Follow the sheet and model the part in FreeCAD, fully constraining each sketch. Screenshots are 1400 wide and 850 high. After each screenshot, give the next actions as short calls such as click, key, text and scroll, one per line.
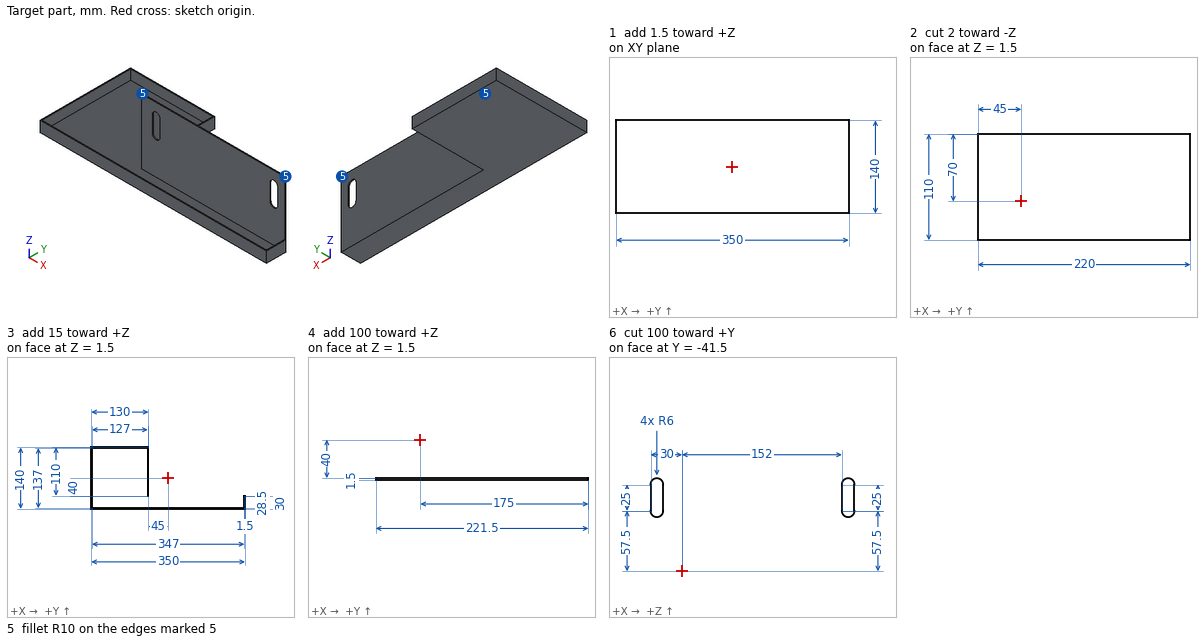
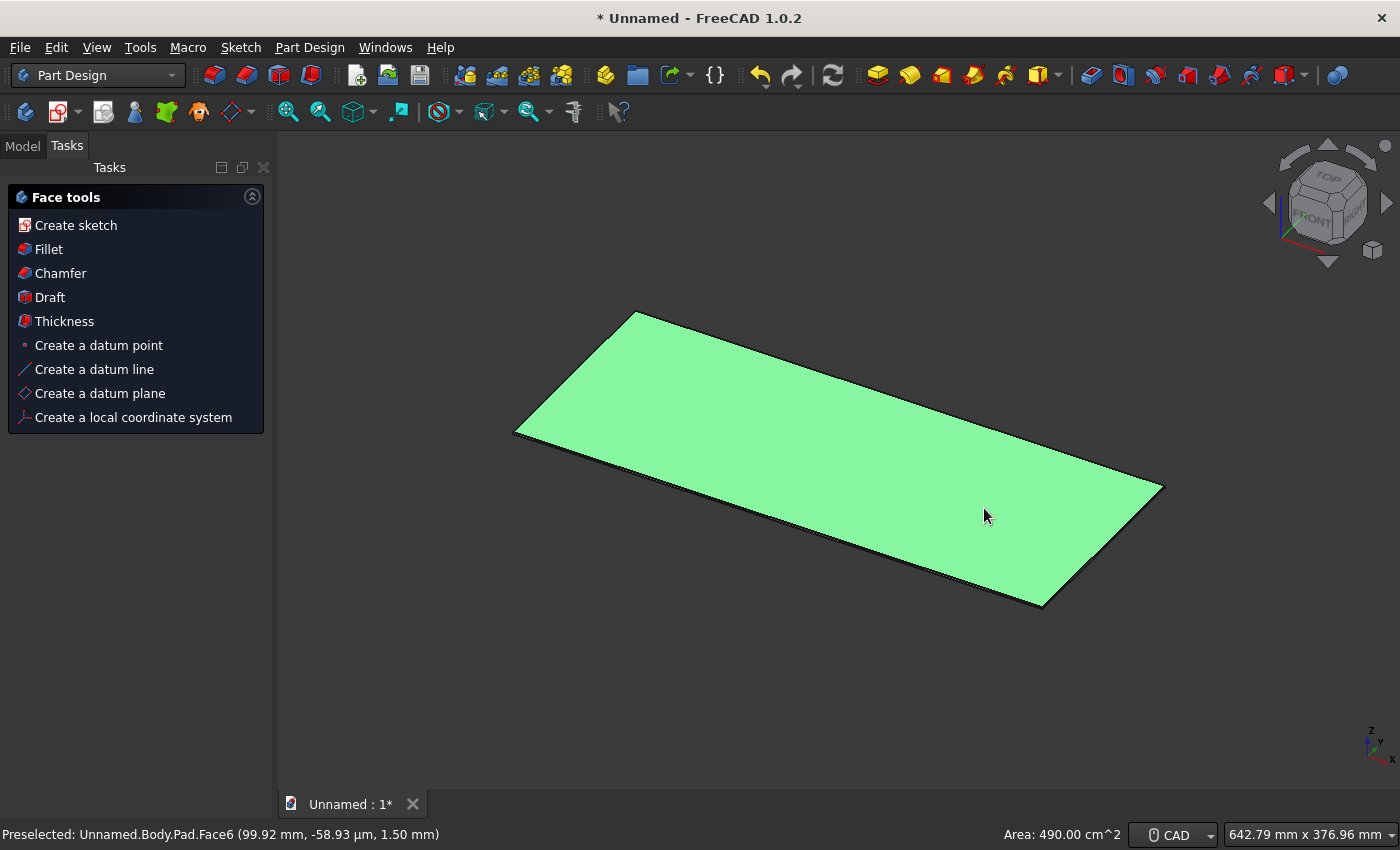
click(58, 112)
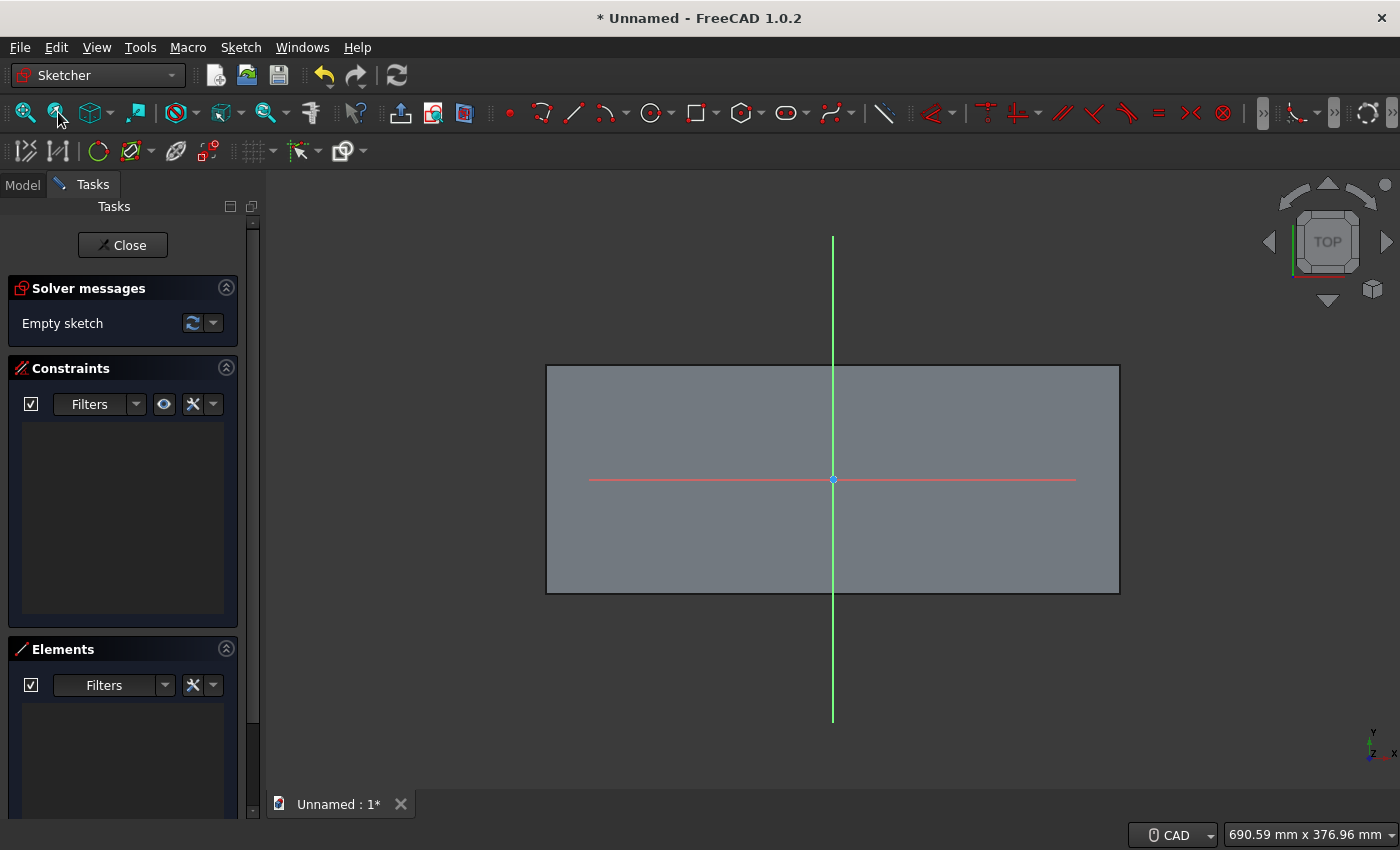
scroll(1153, 425, up, 3)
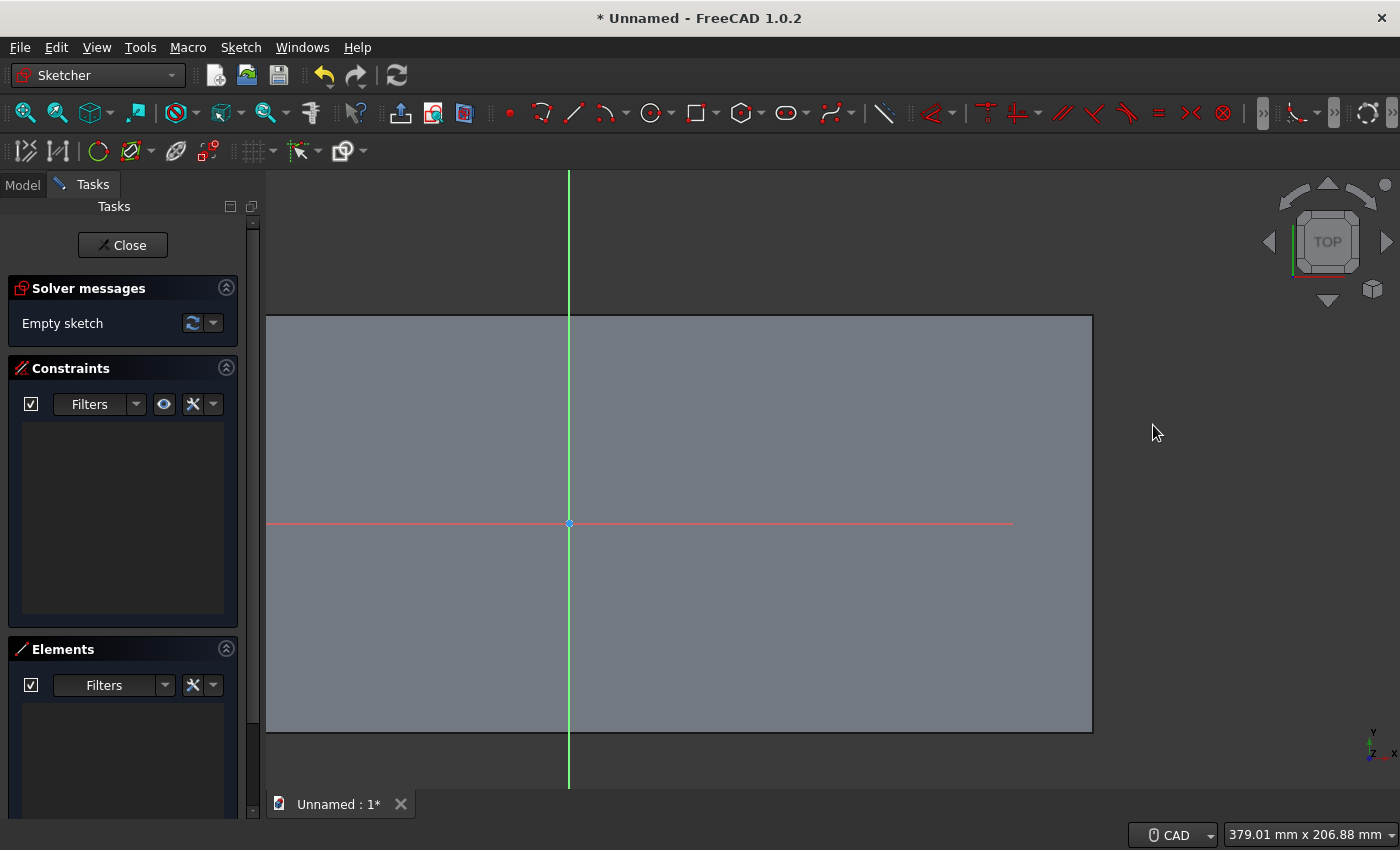
click(696, 114)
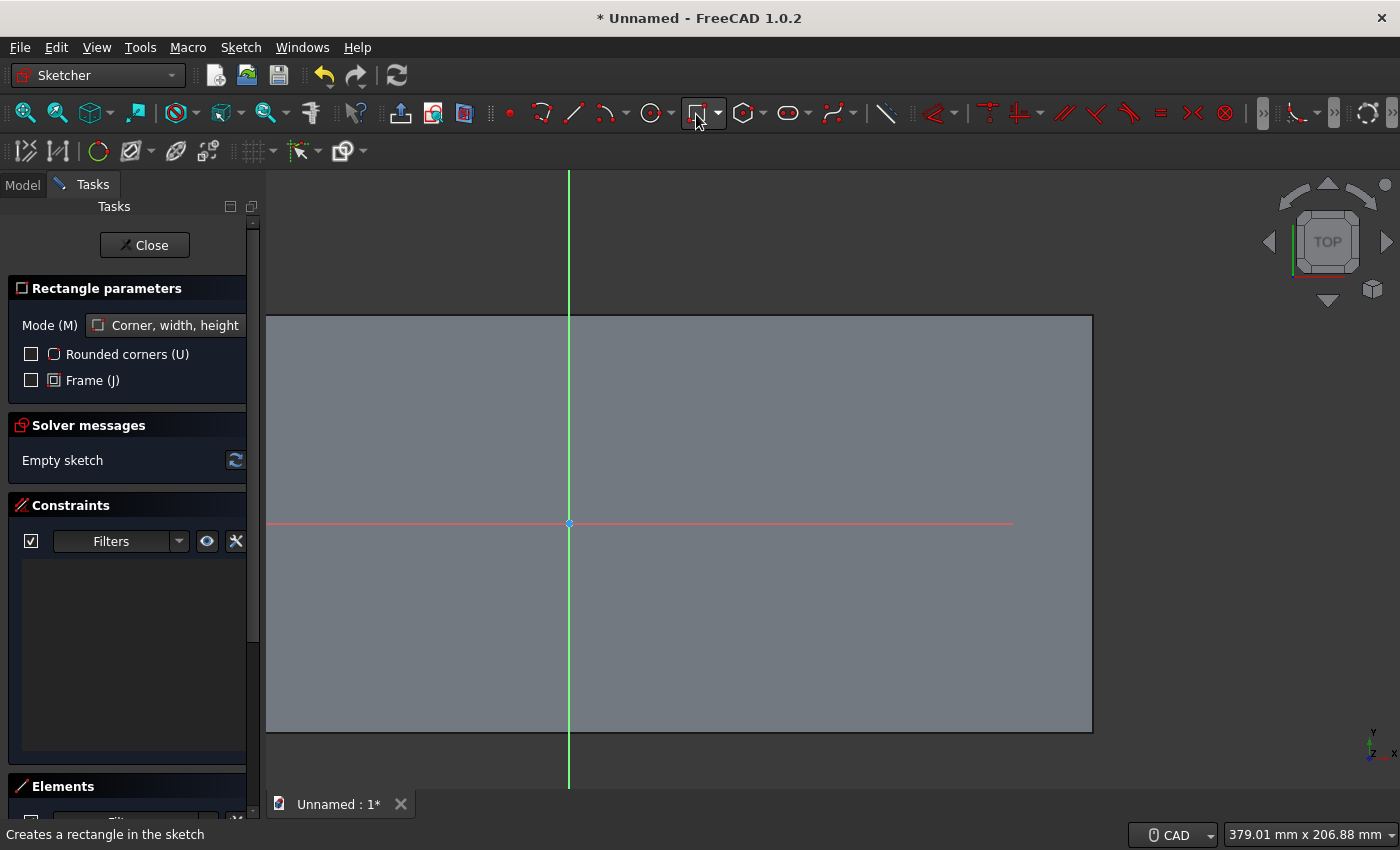
click(435, 315)
click(1093, 644)
key(Escape)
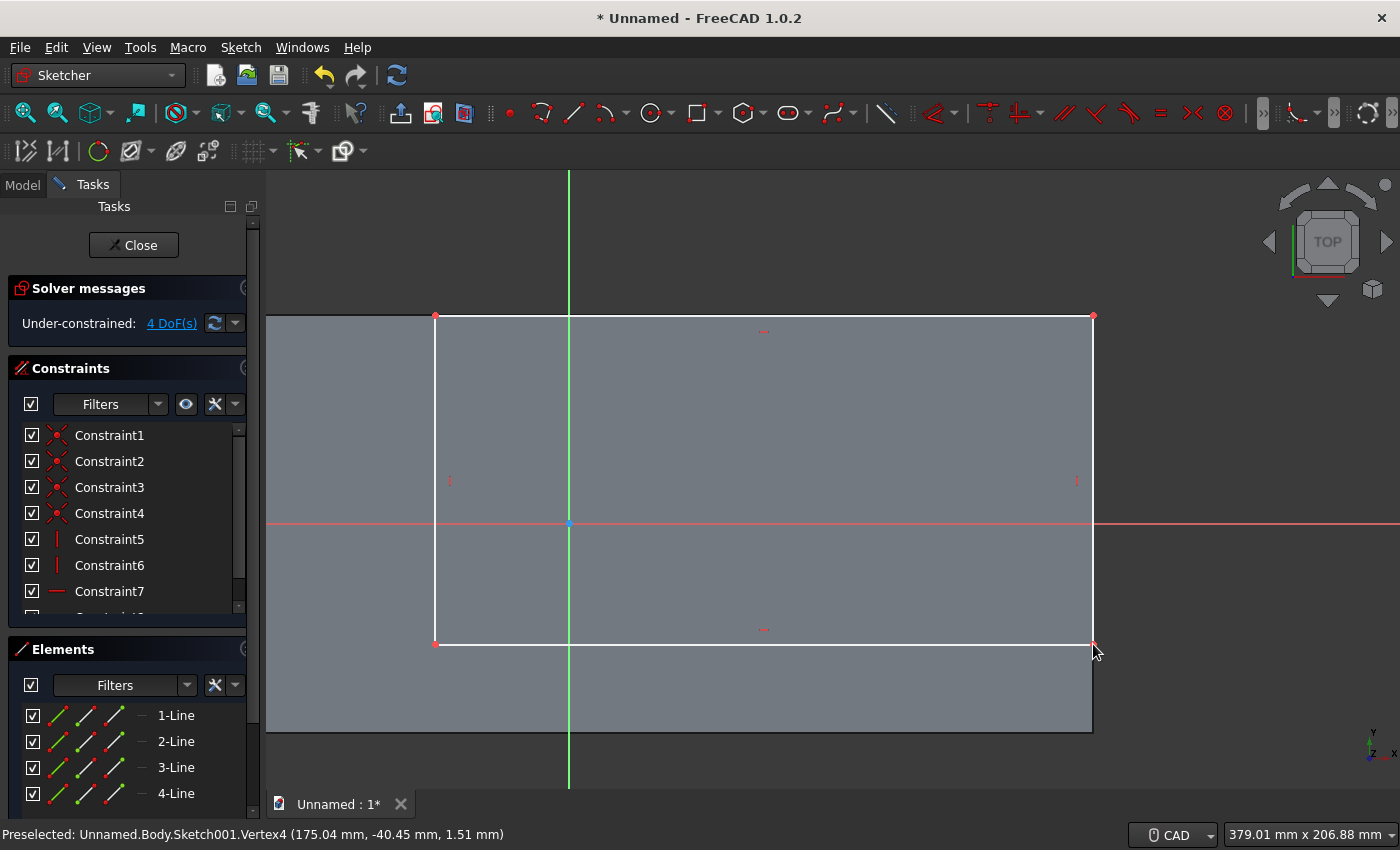
click(934, 114)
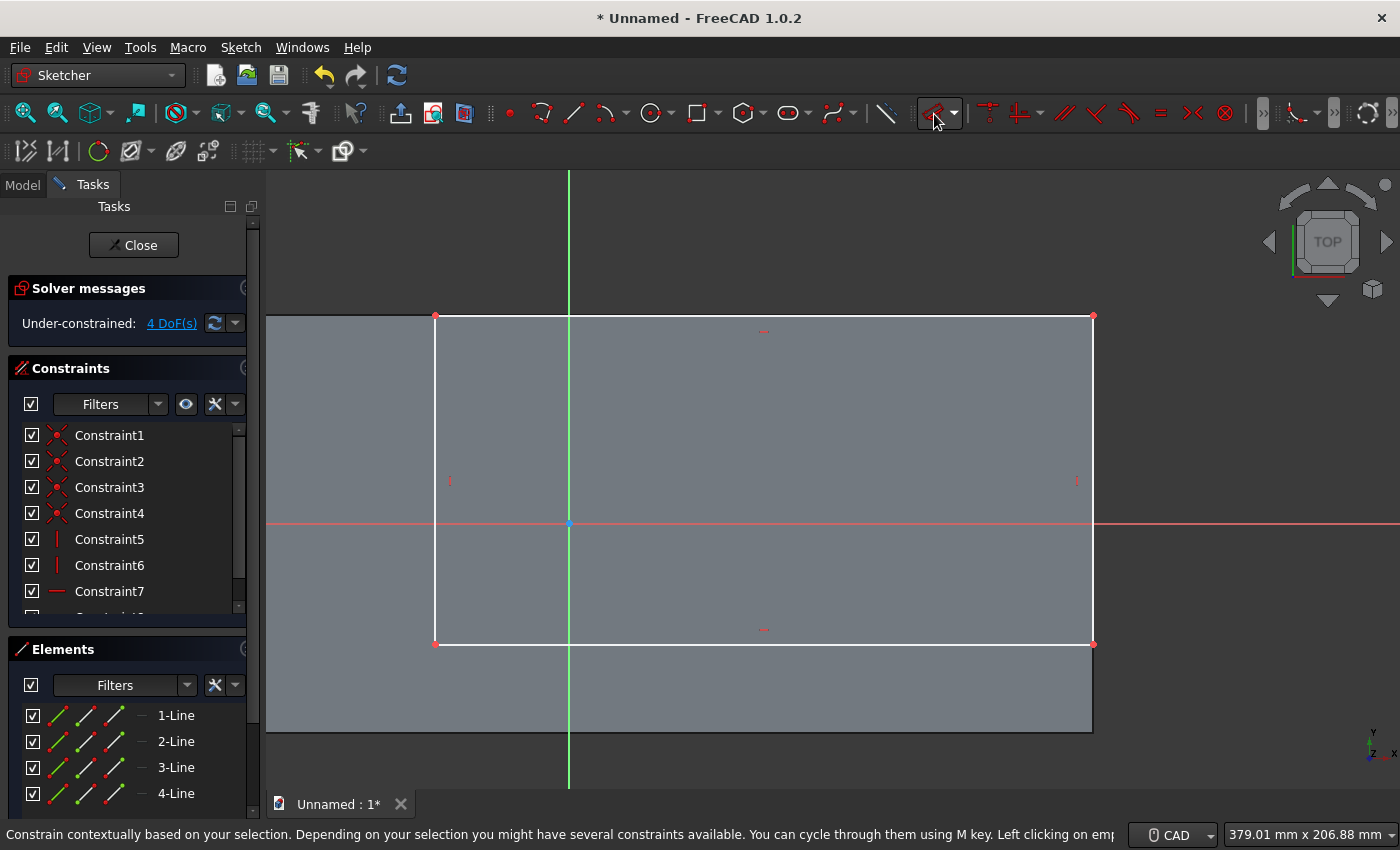
click(435, 415)
click(401, 481)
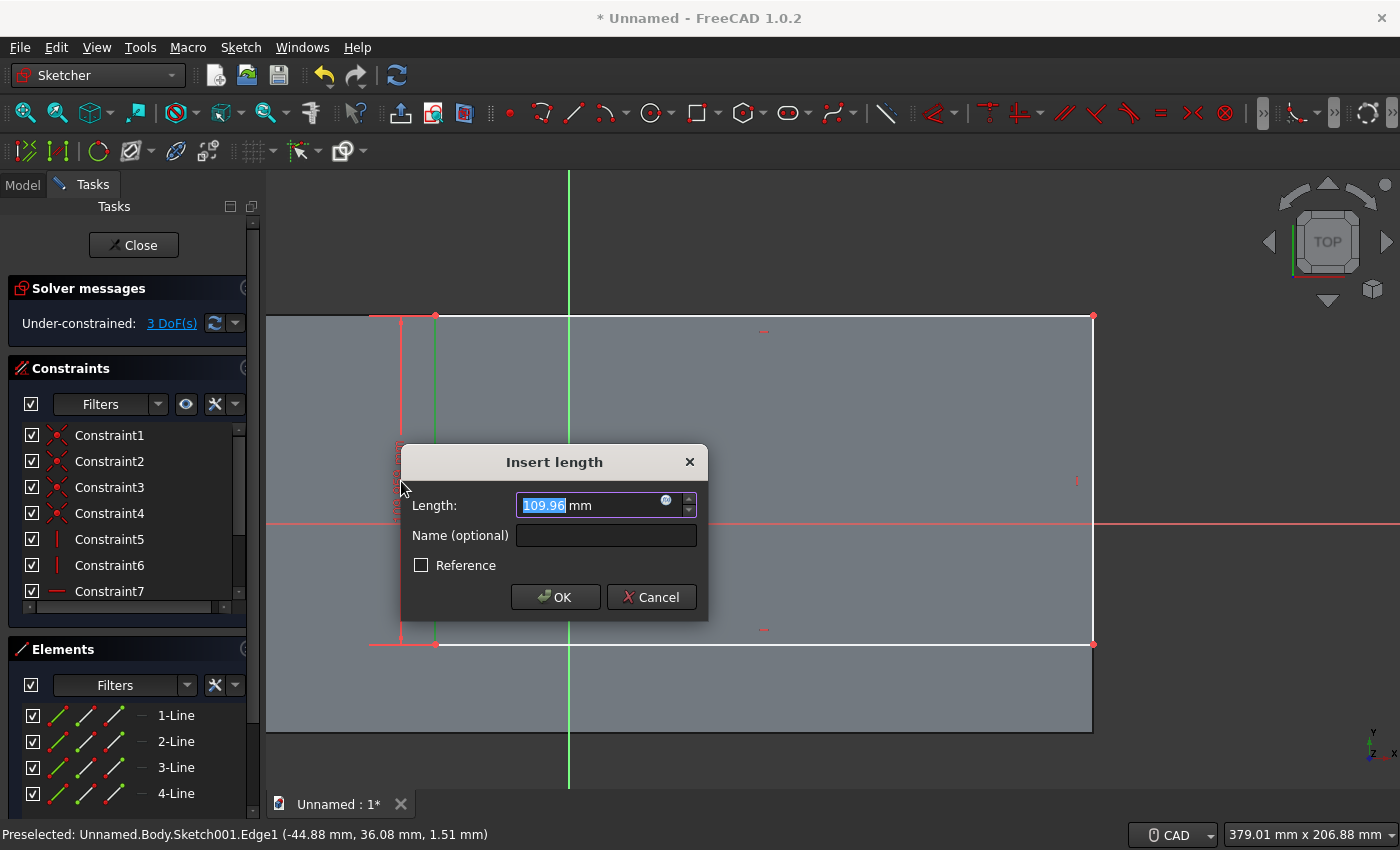
text(110)
key(Return)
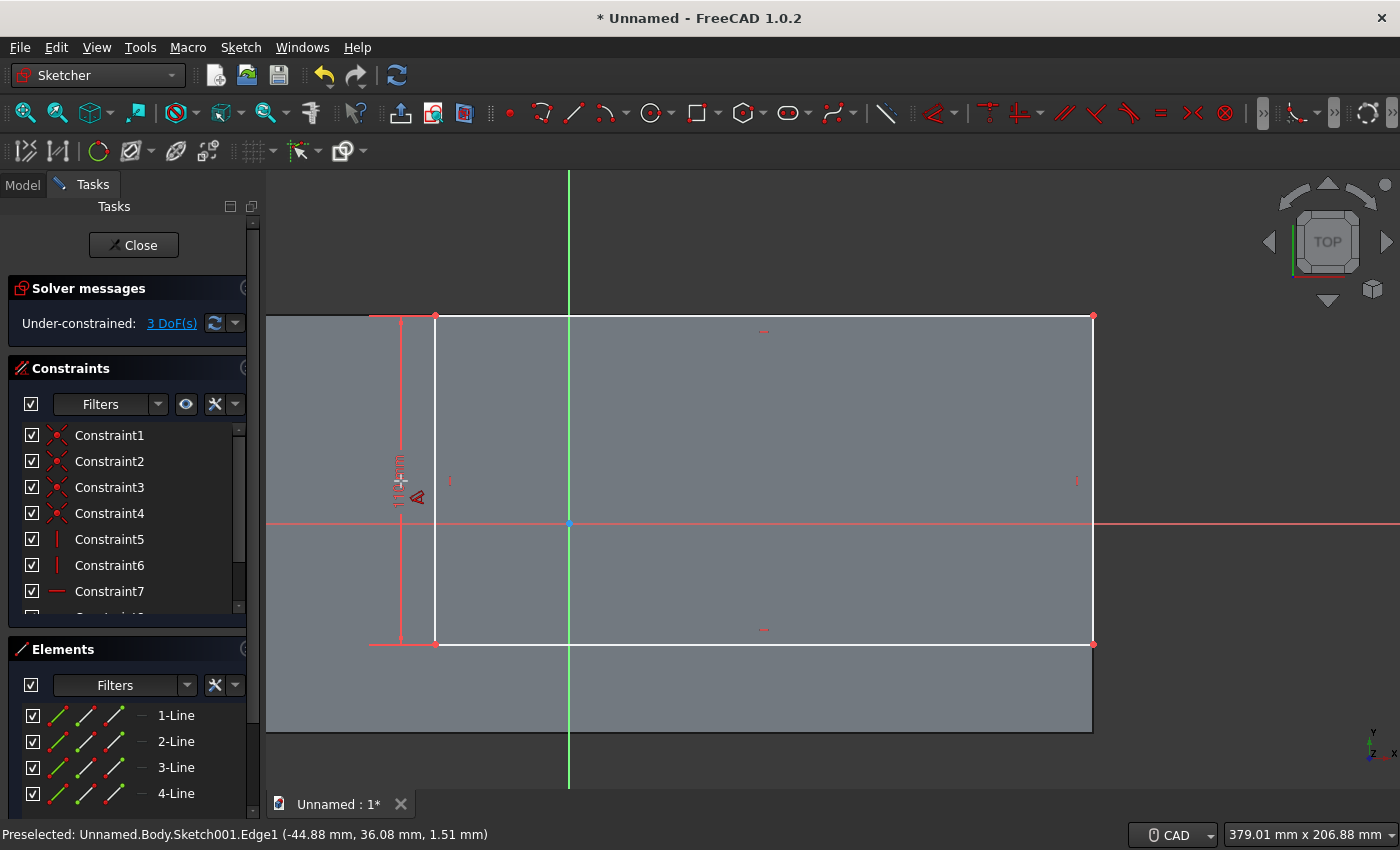
click(632, 645)
click(764, 679)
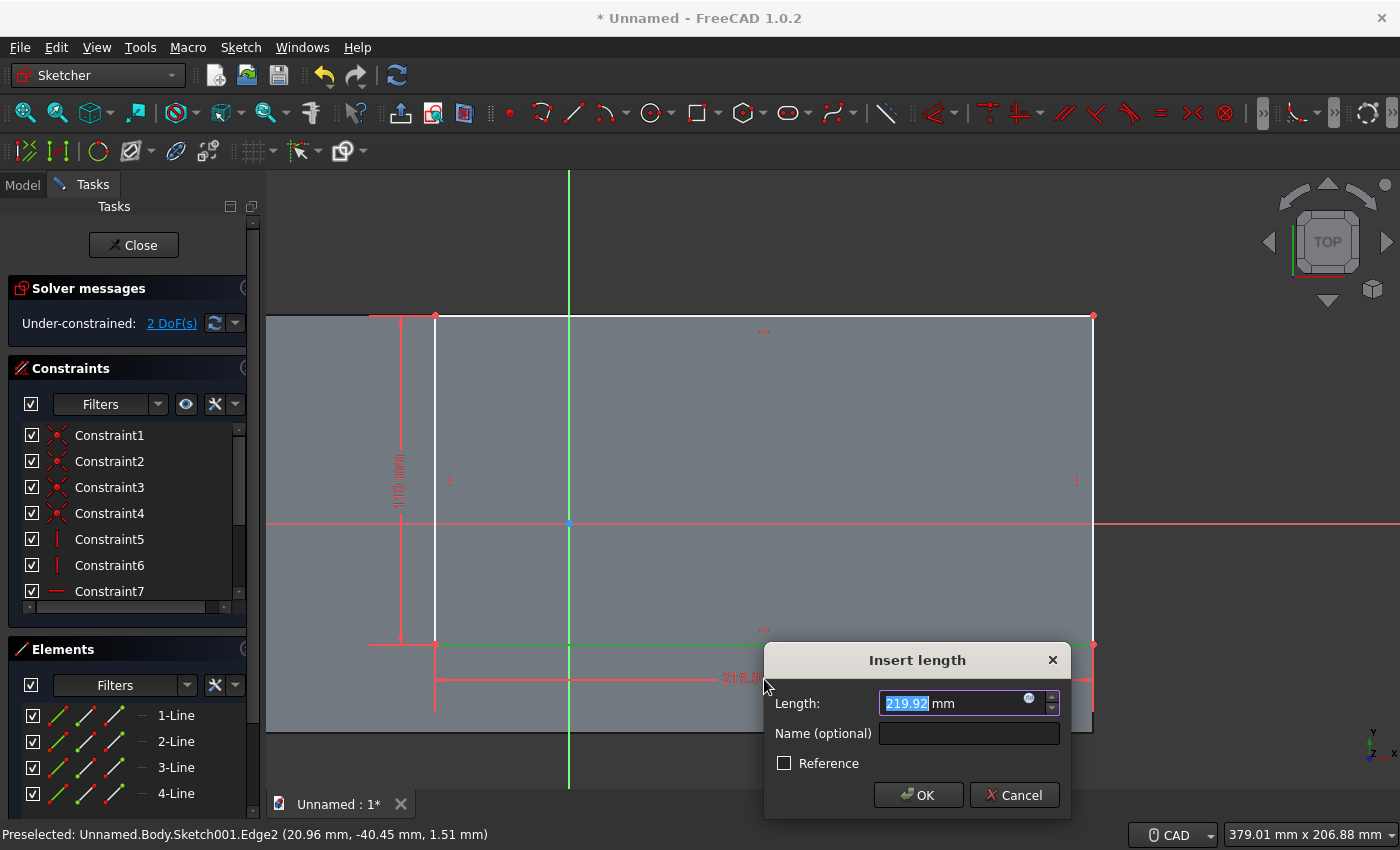
text(220)
key(Return)